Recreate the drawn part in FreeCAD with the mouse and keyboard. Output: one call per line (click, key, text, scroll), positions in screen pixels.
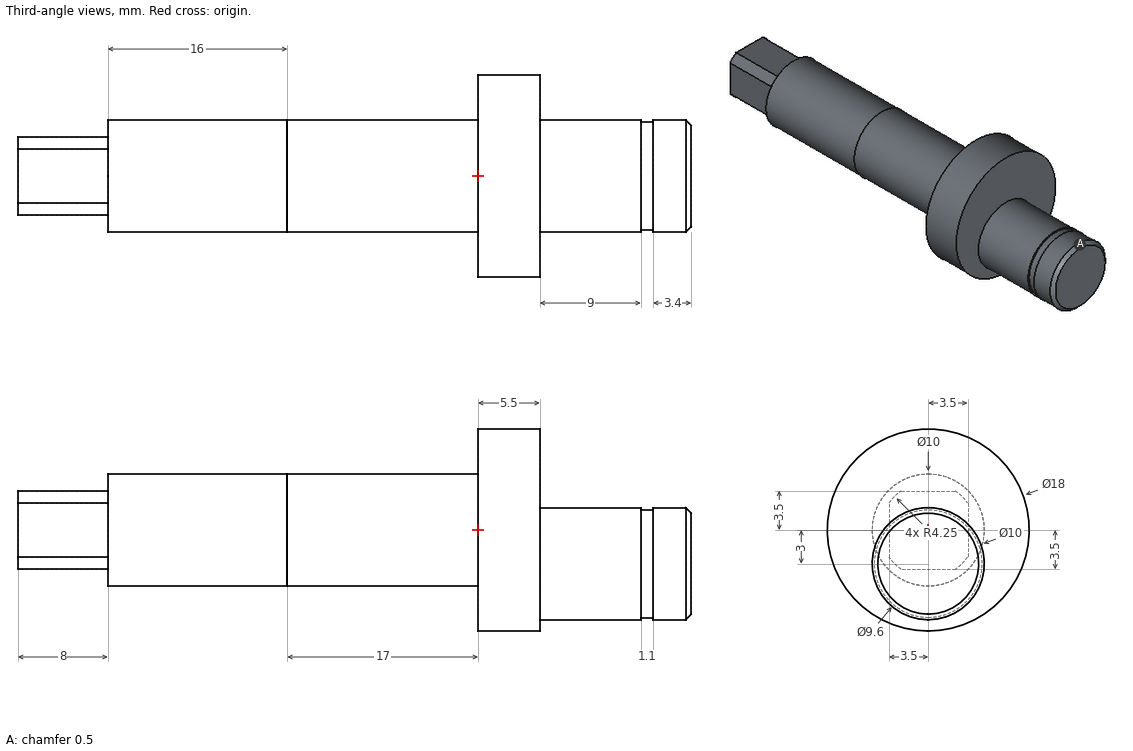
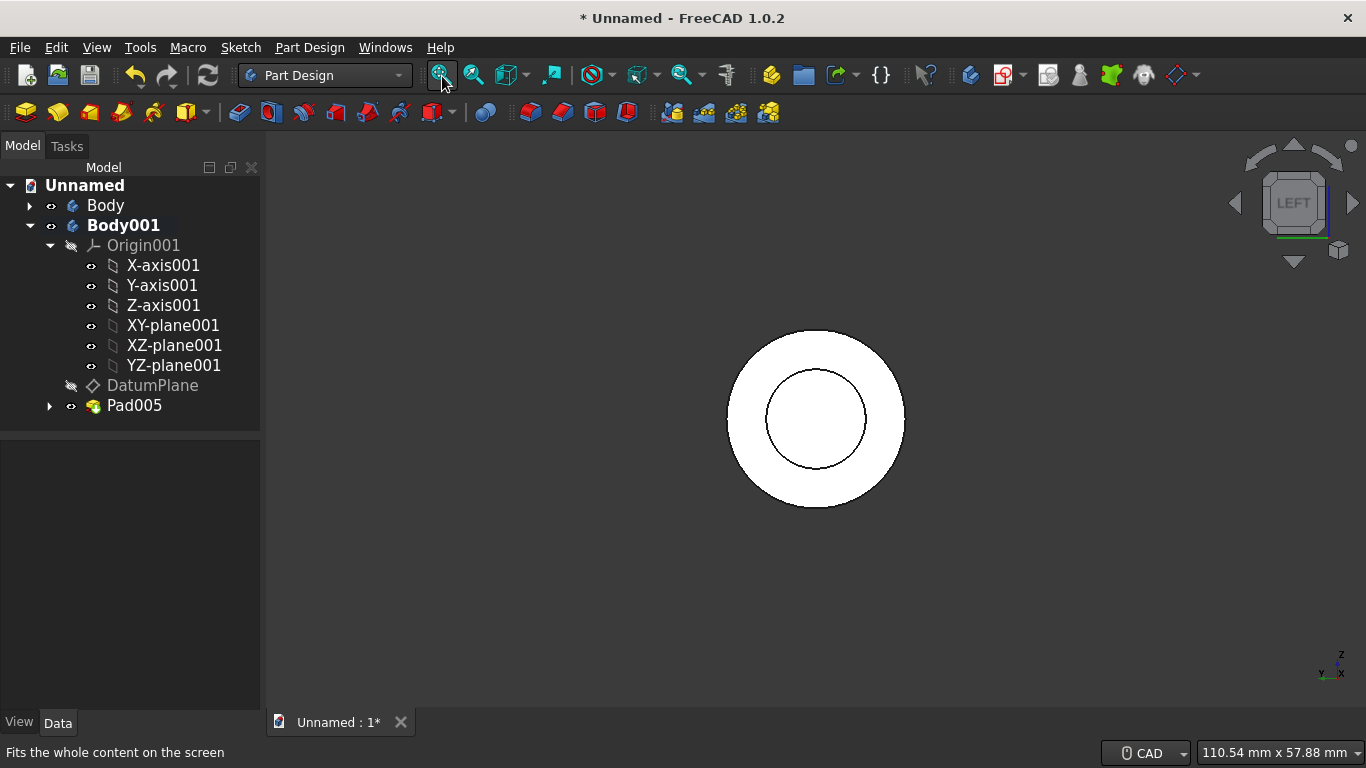
click(816, 418)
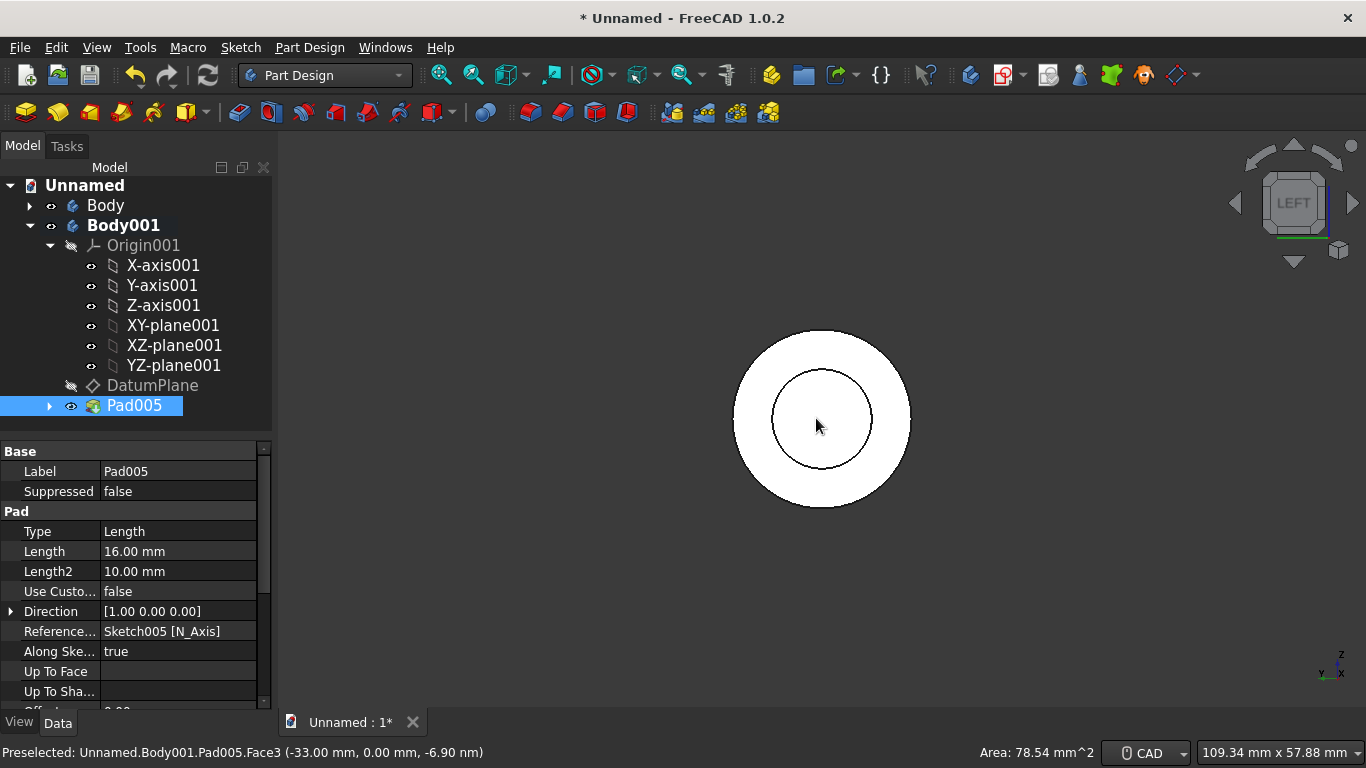
click(1004, 76)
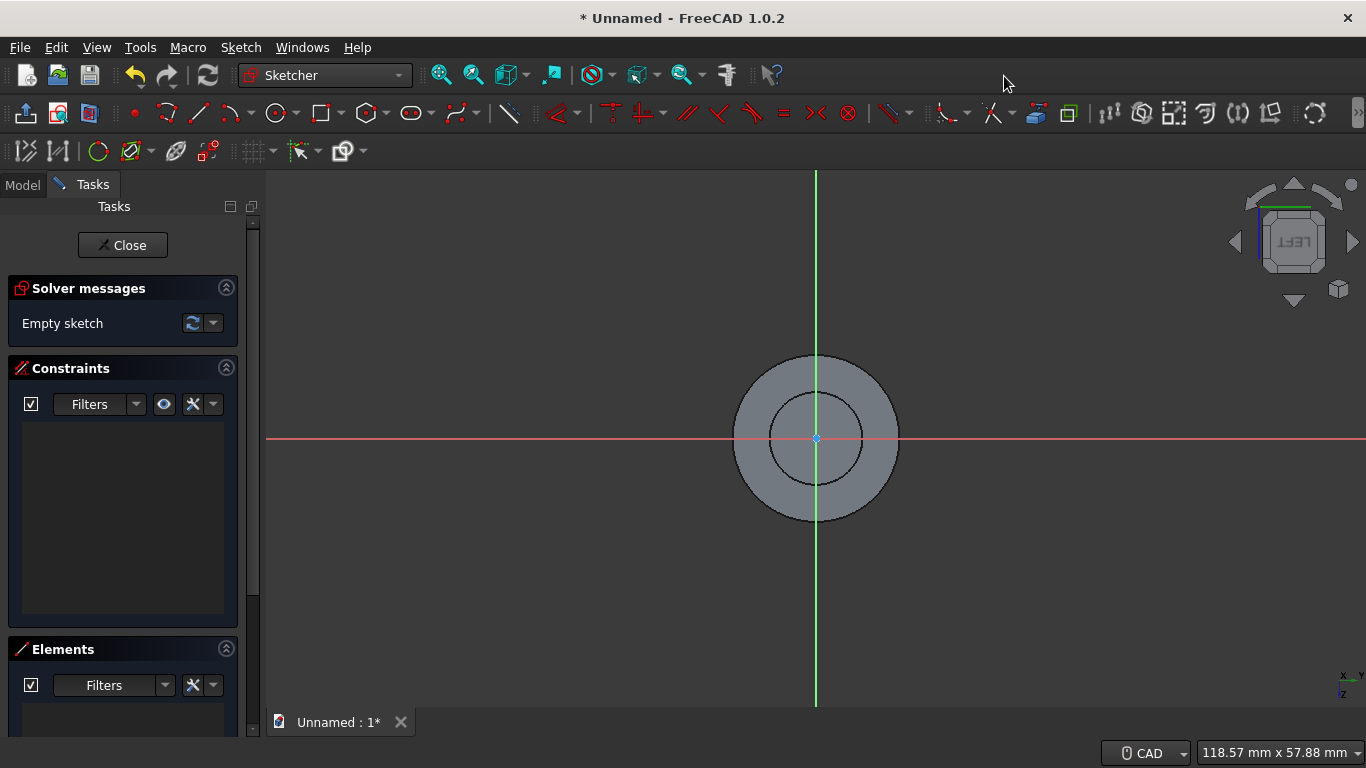
scroll(833, 438, up, 8)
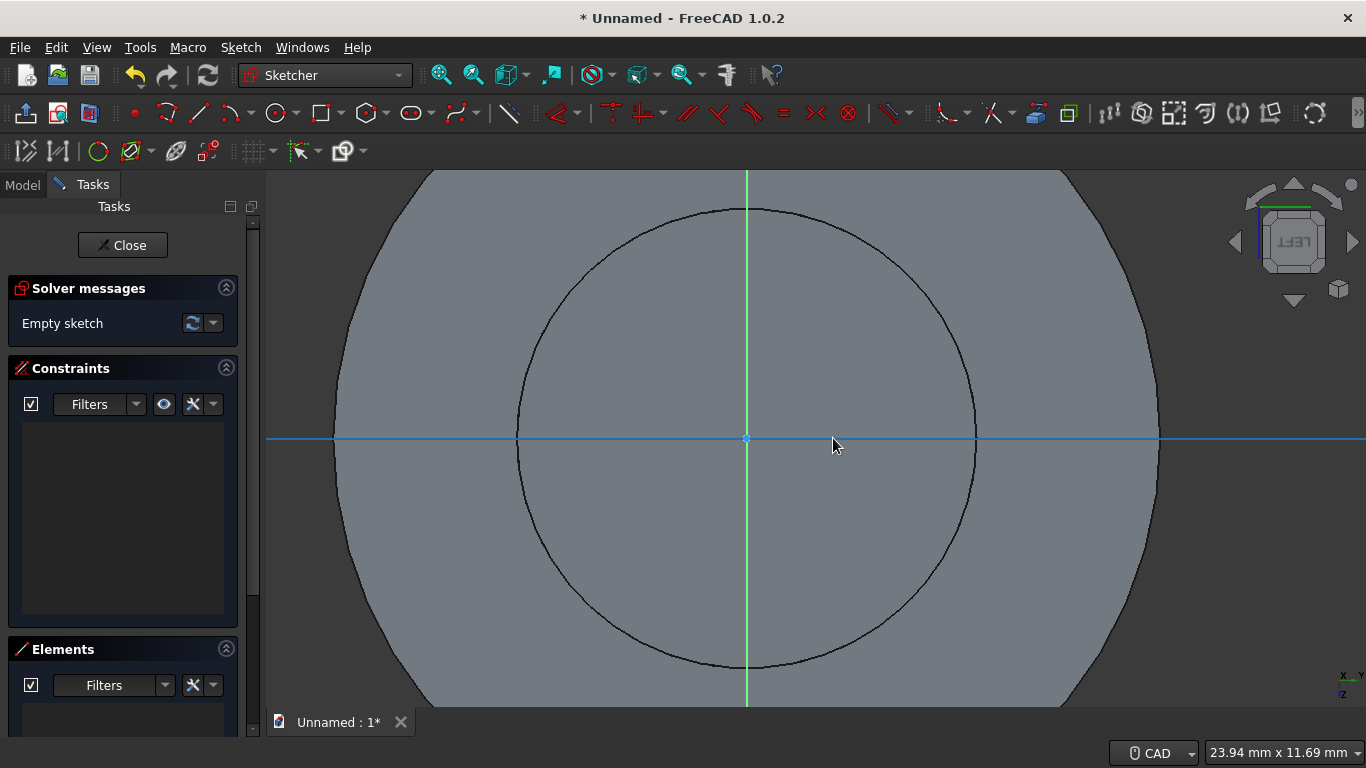
key(g)
key(l)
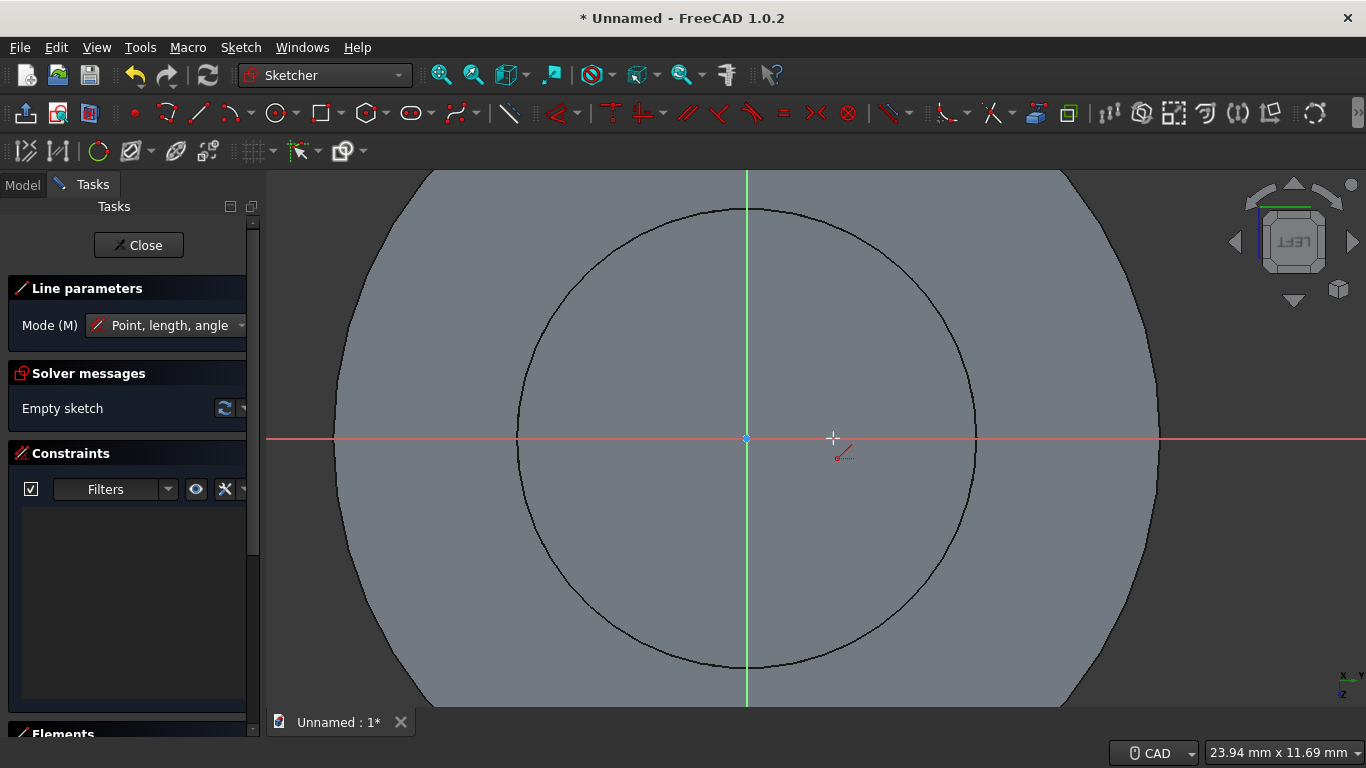
click(586, 328)
click(586, 549)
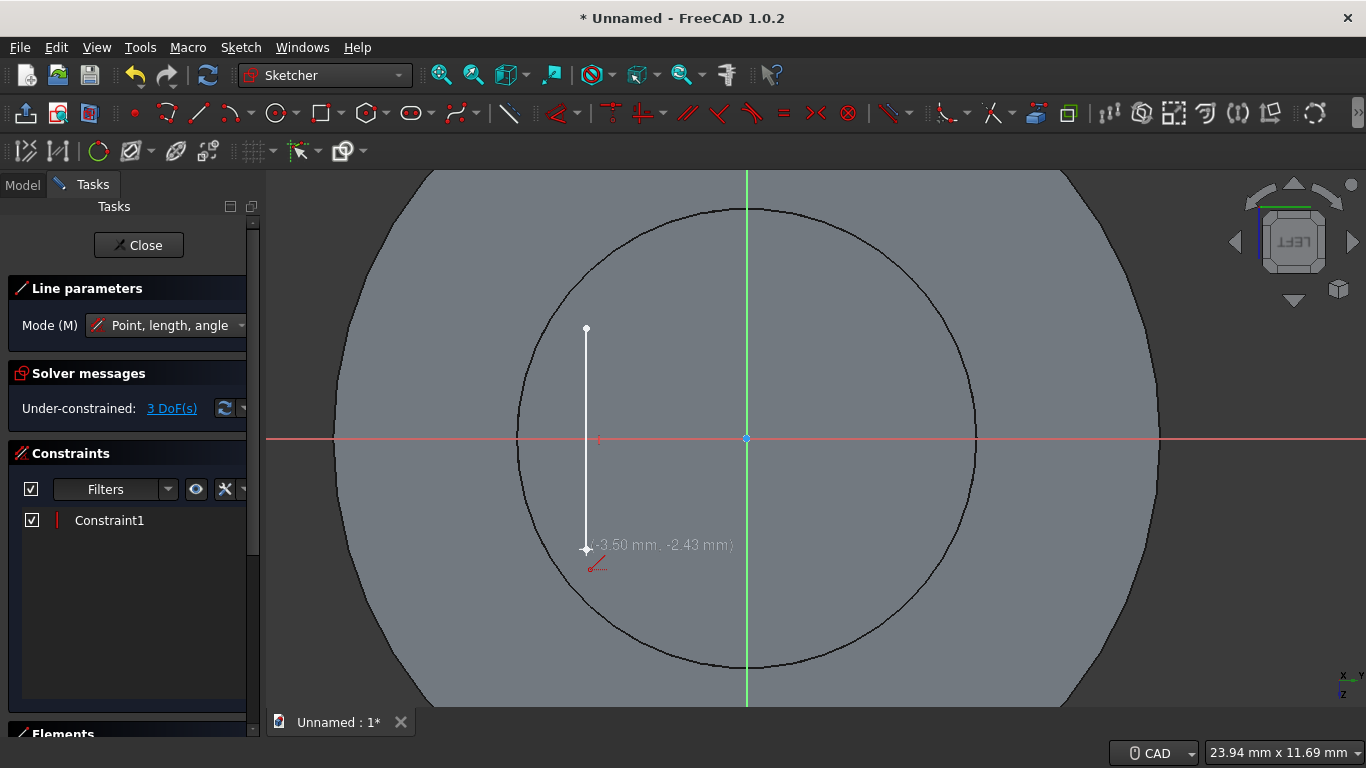
click(636, 599)
click(858, 599)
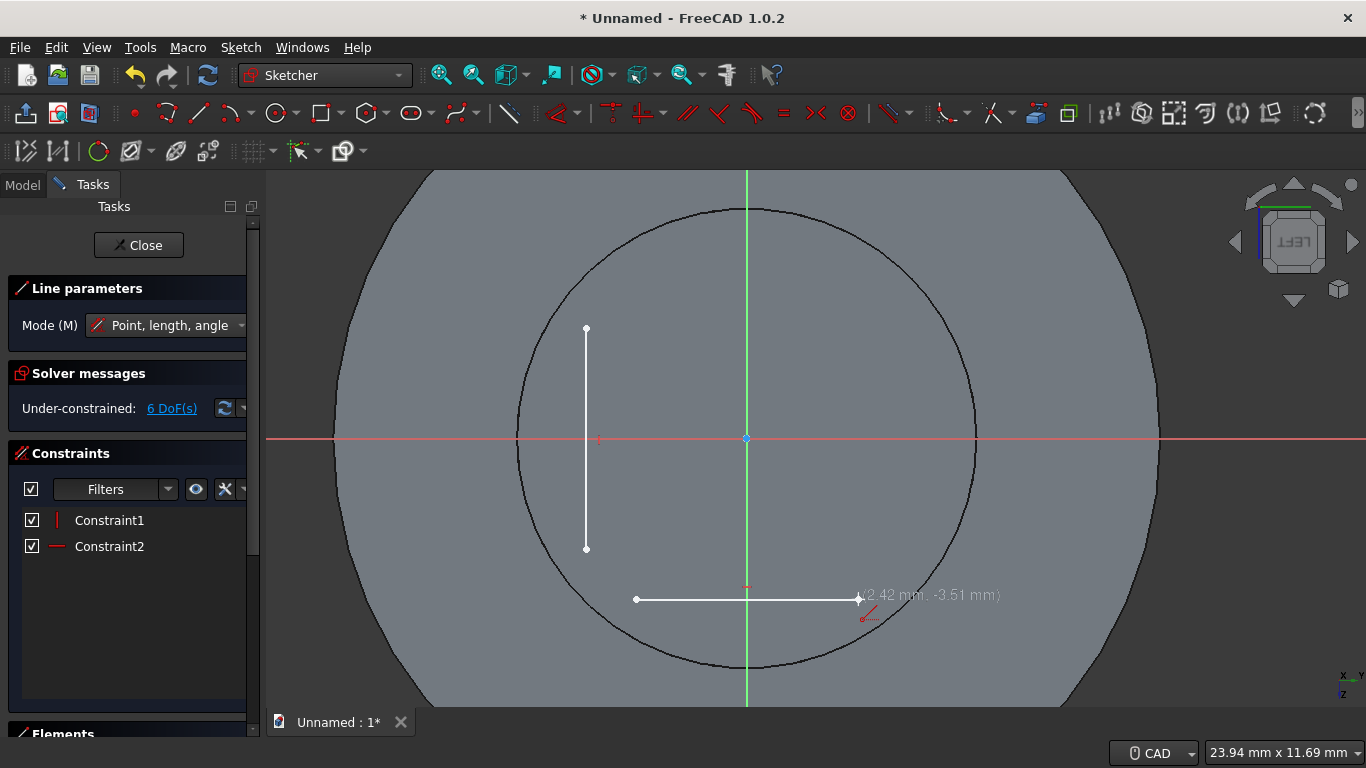
click(908, 549)
click(908, 328)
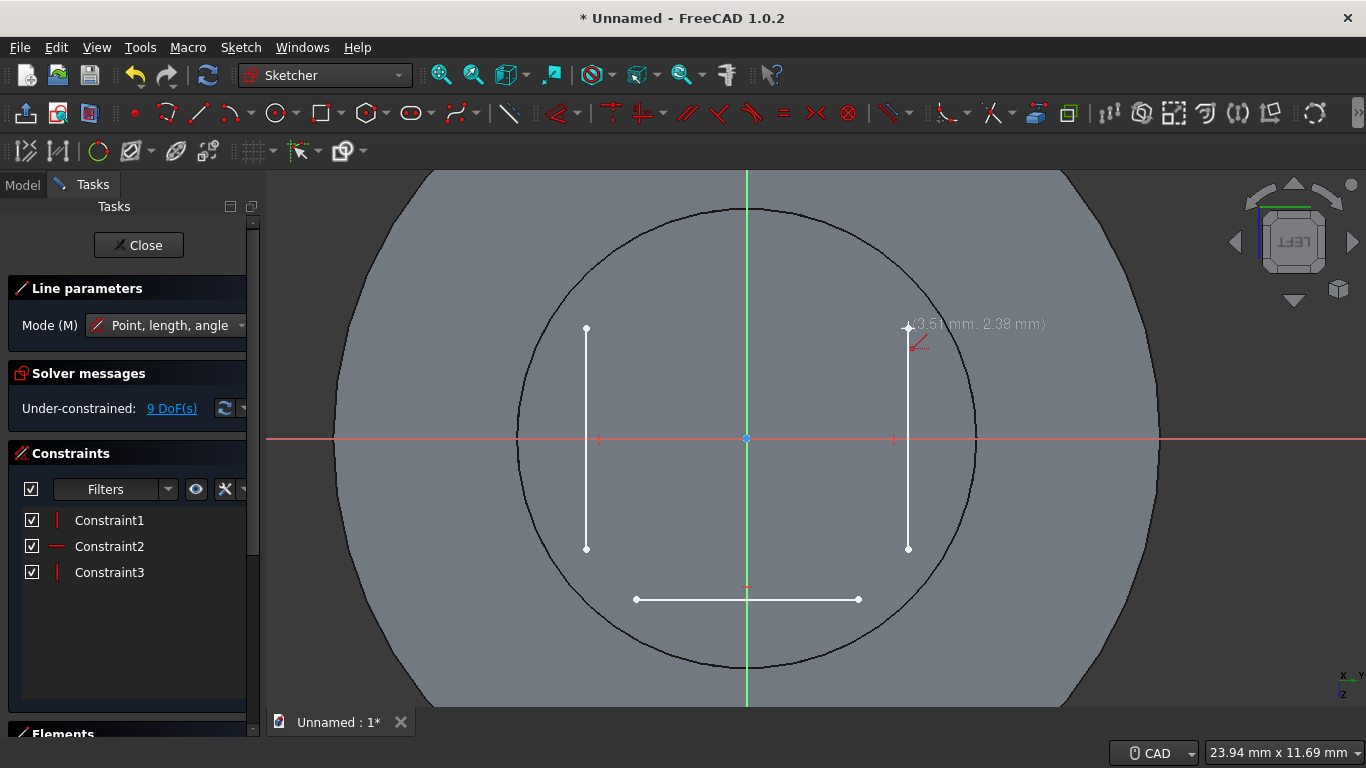
click(858, 278)
click(636, 278)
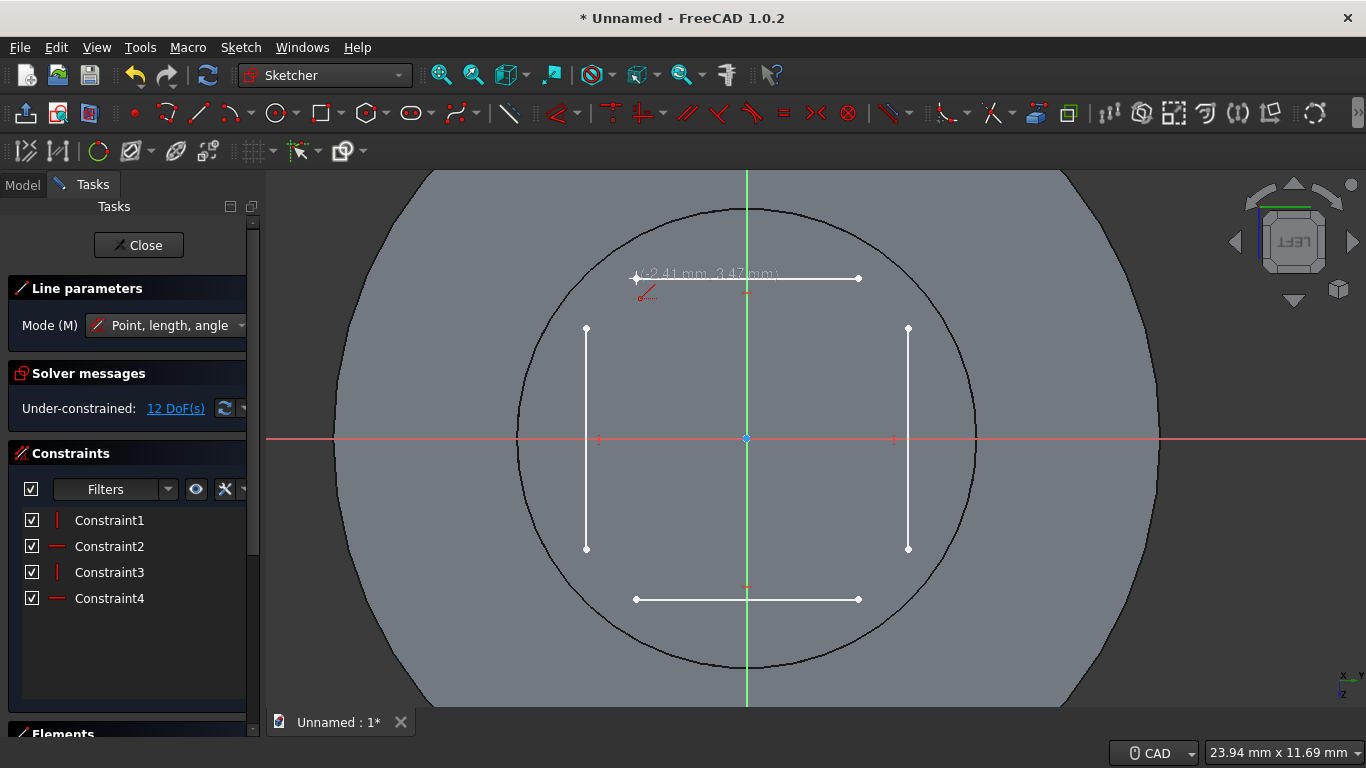
key(g)
key(3)
key(a)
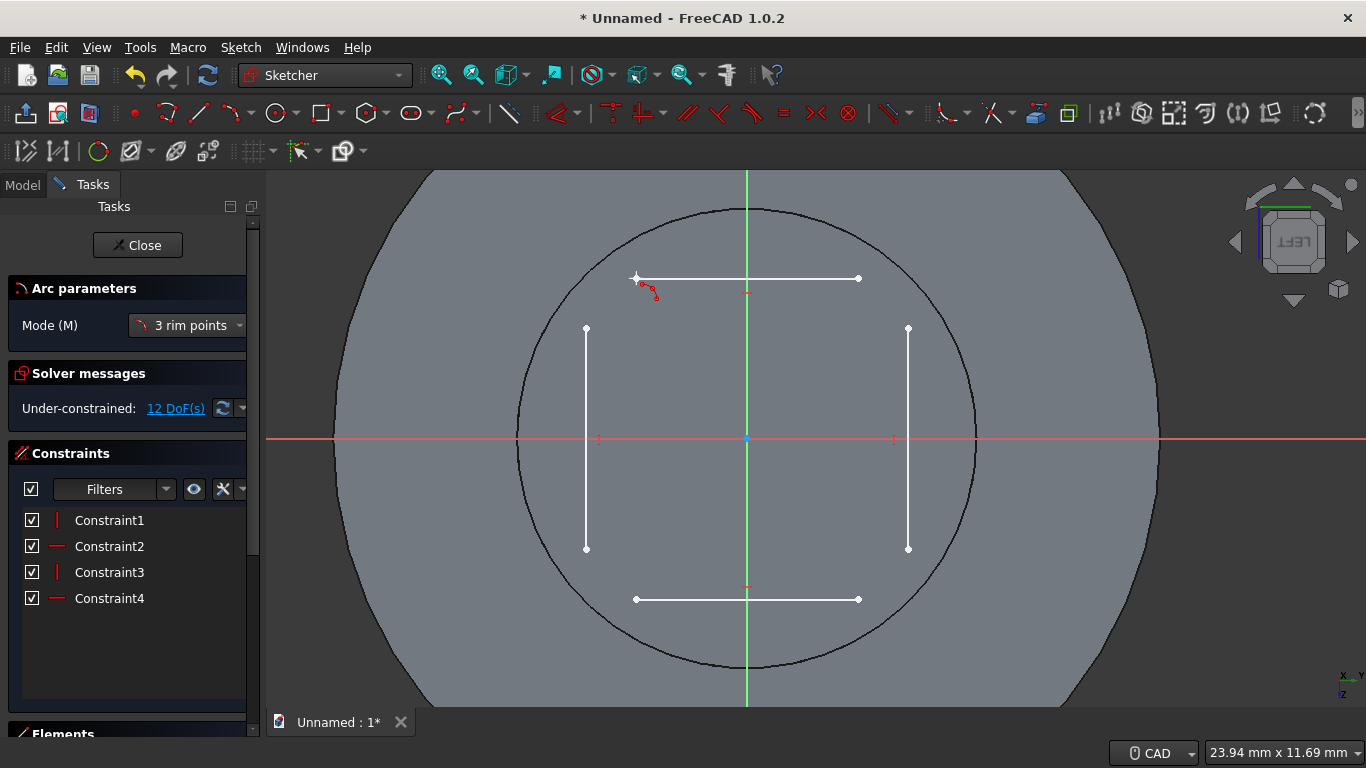
click(586, 550)
click(636, 600)